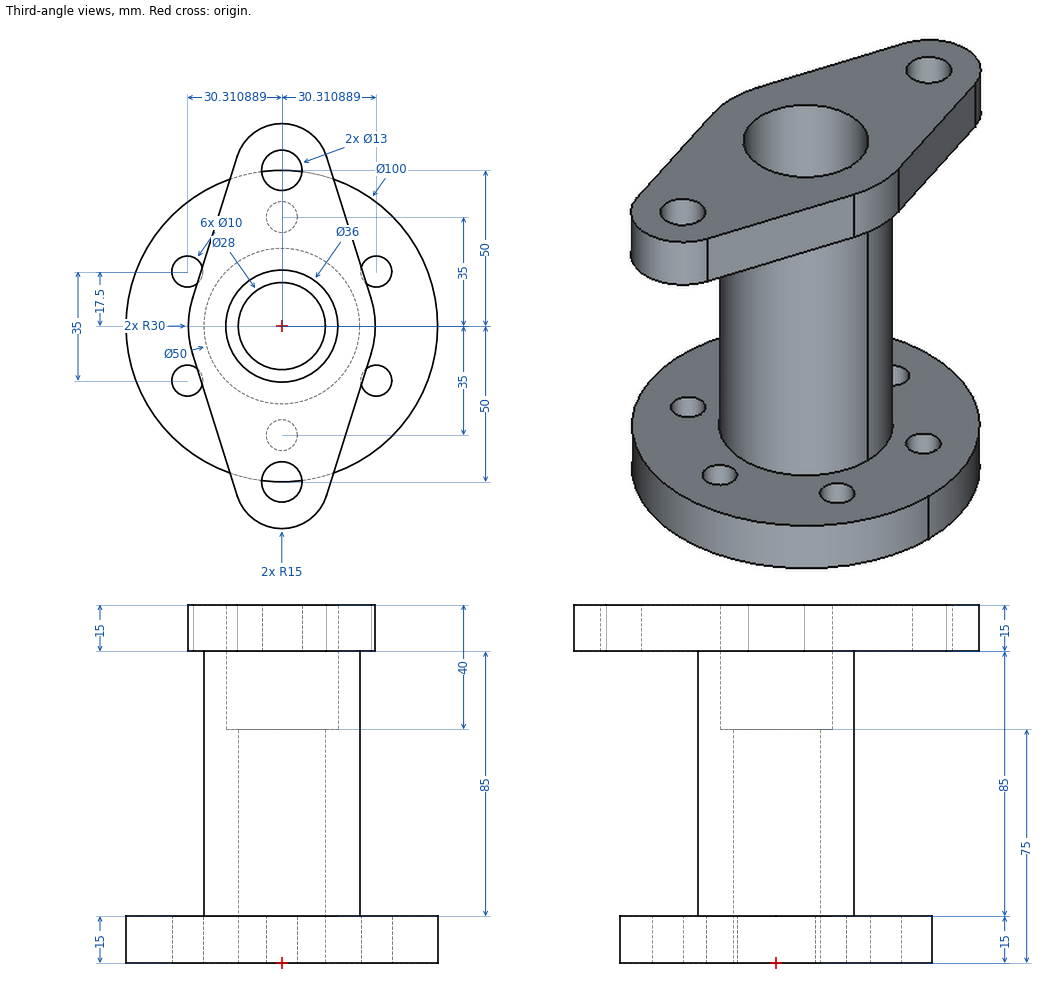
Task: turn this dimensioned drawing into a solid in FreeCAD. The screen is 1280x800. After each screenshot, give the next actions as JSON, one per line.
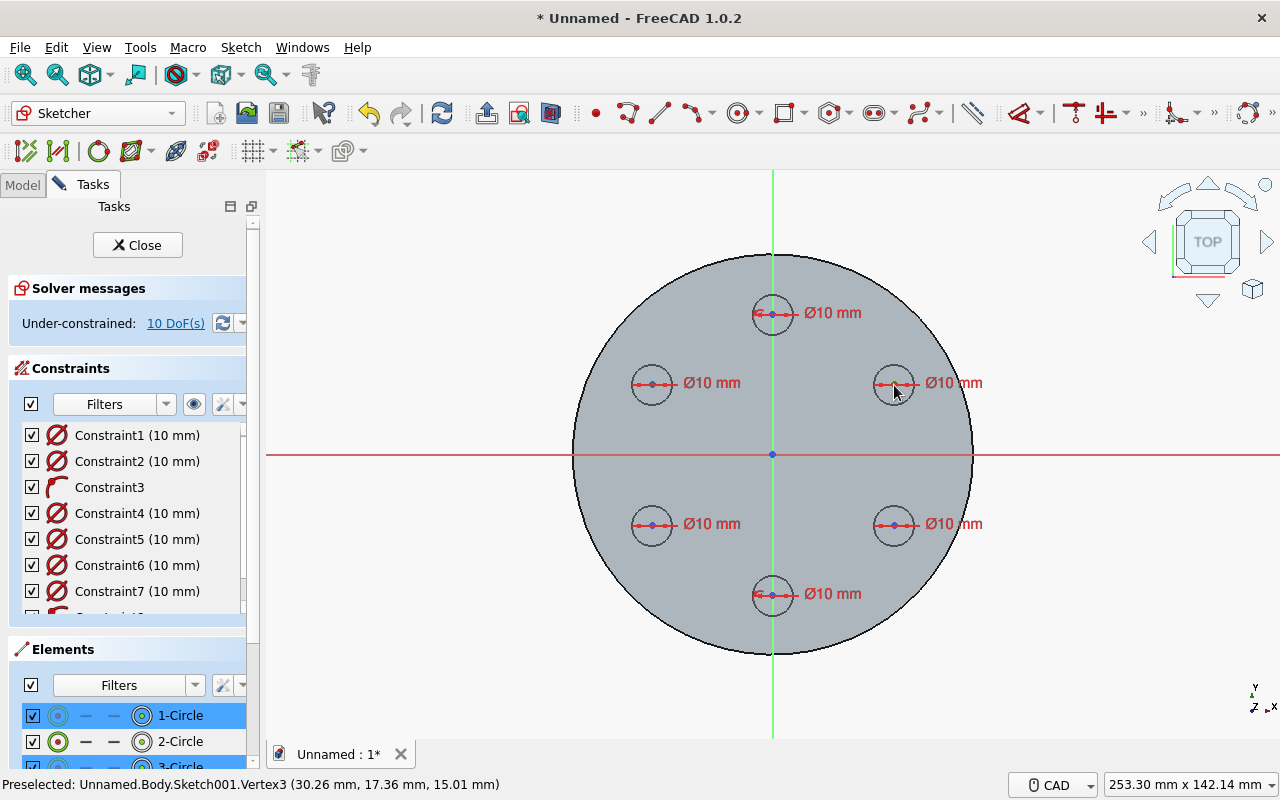
{"action": "key", "text": "h"}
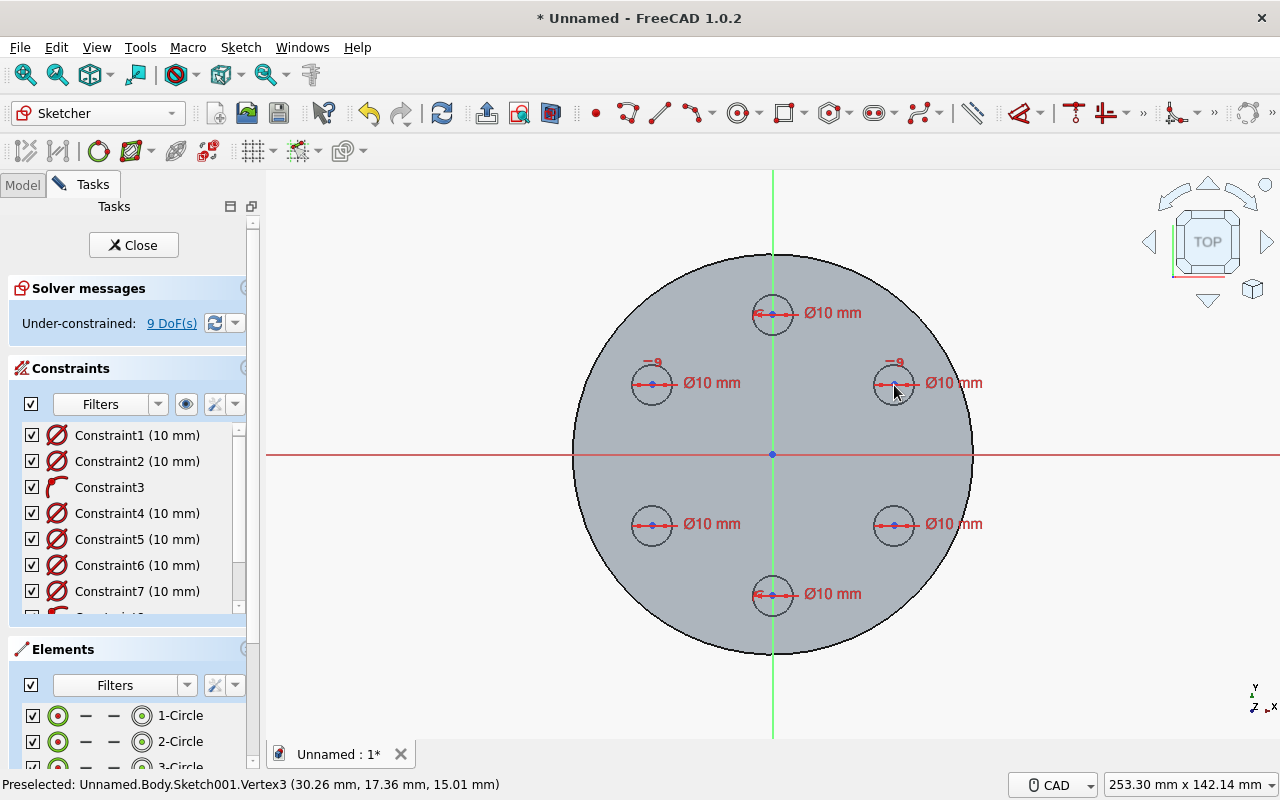
{"action": "left_click", "coordinate": [652, 385]}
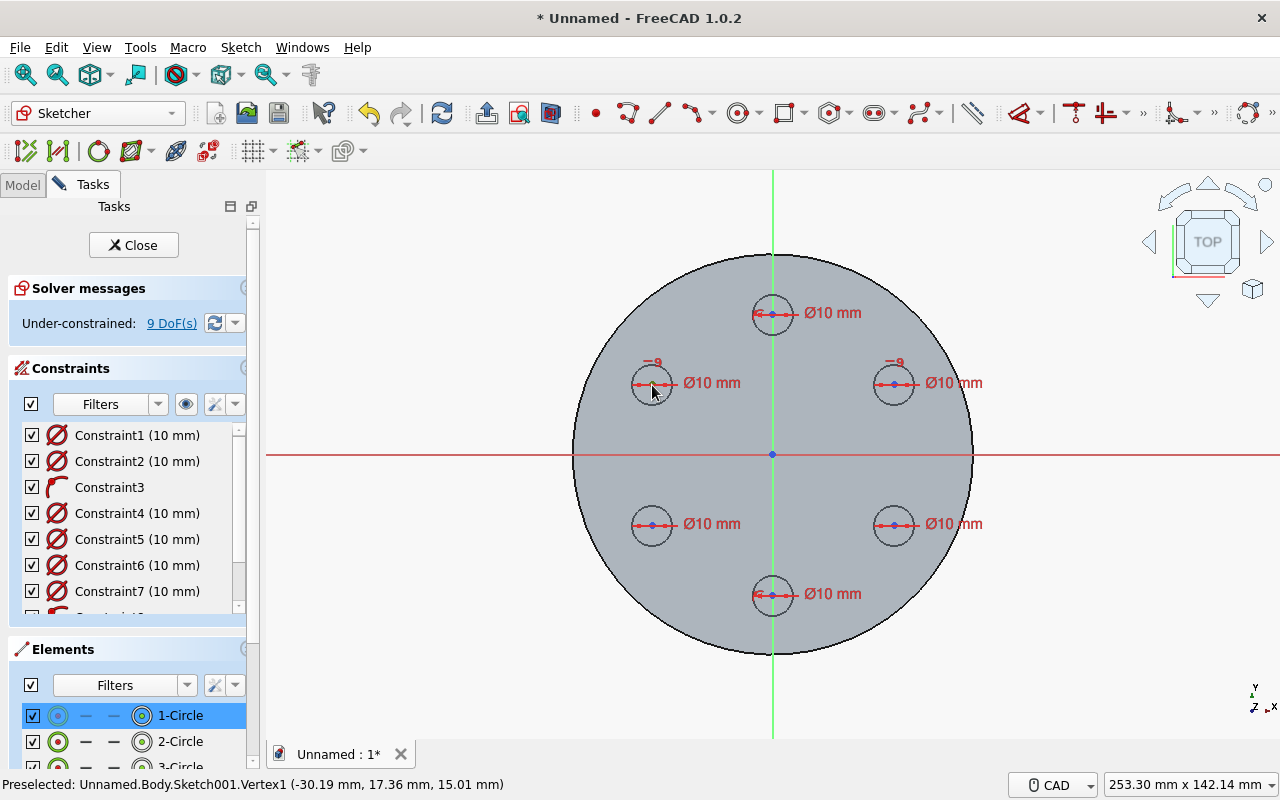
{"action": "left_click", "coordinate": [652, 526]}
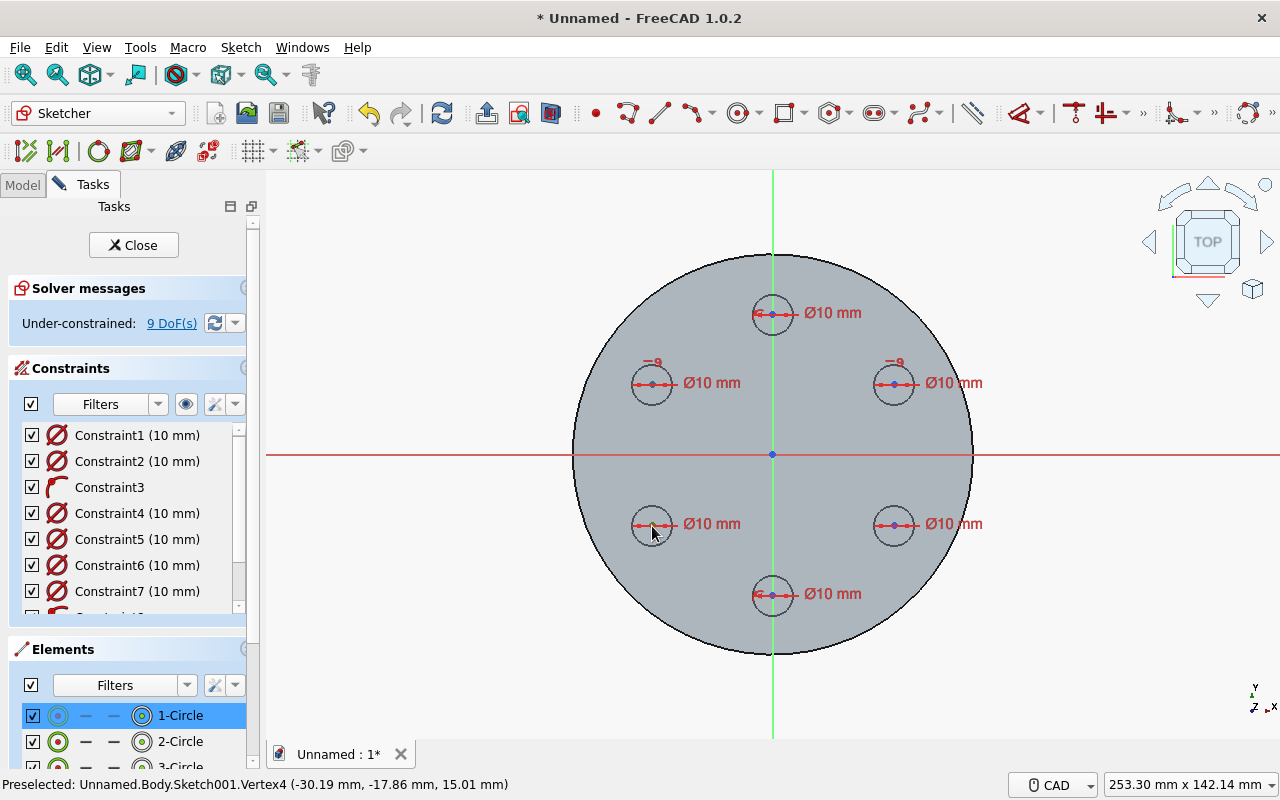
{"action": "key", "text": "v"}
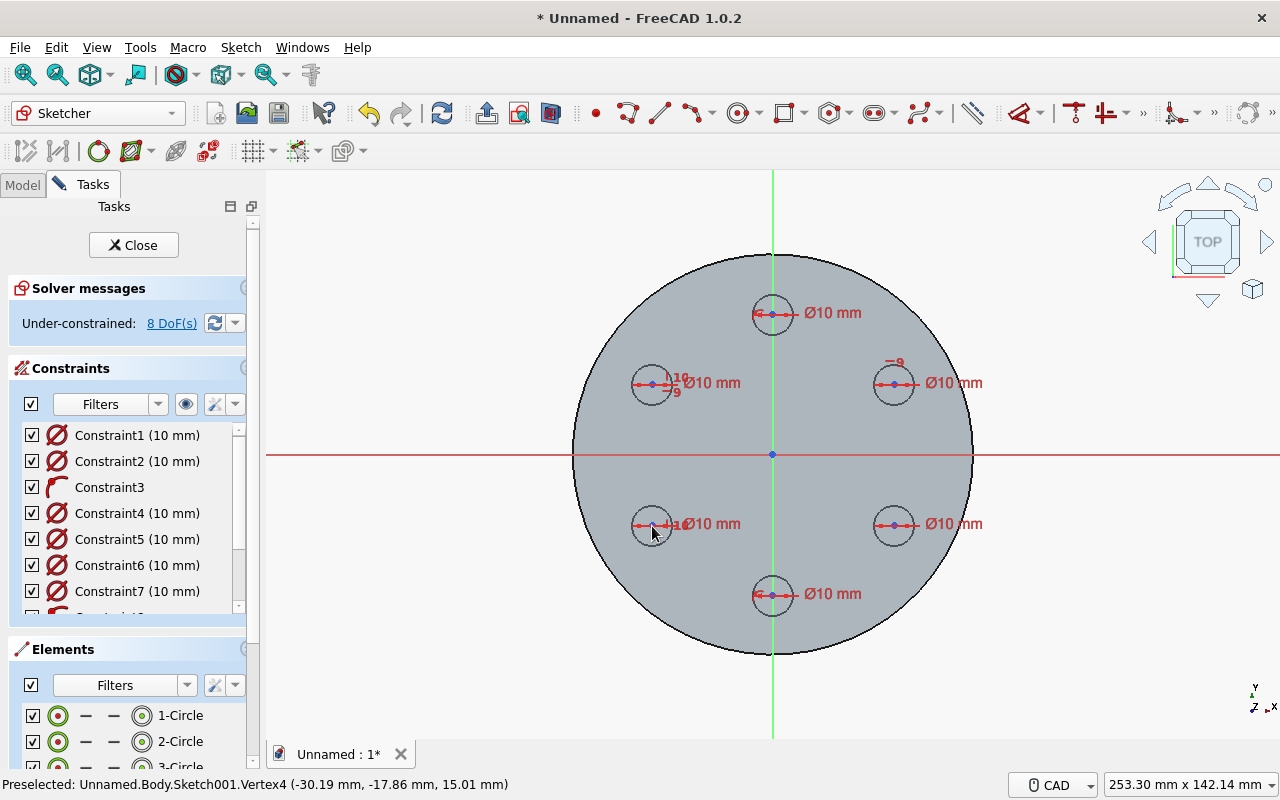
{"action": "left_click", "coordinate": [894, 385]}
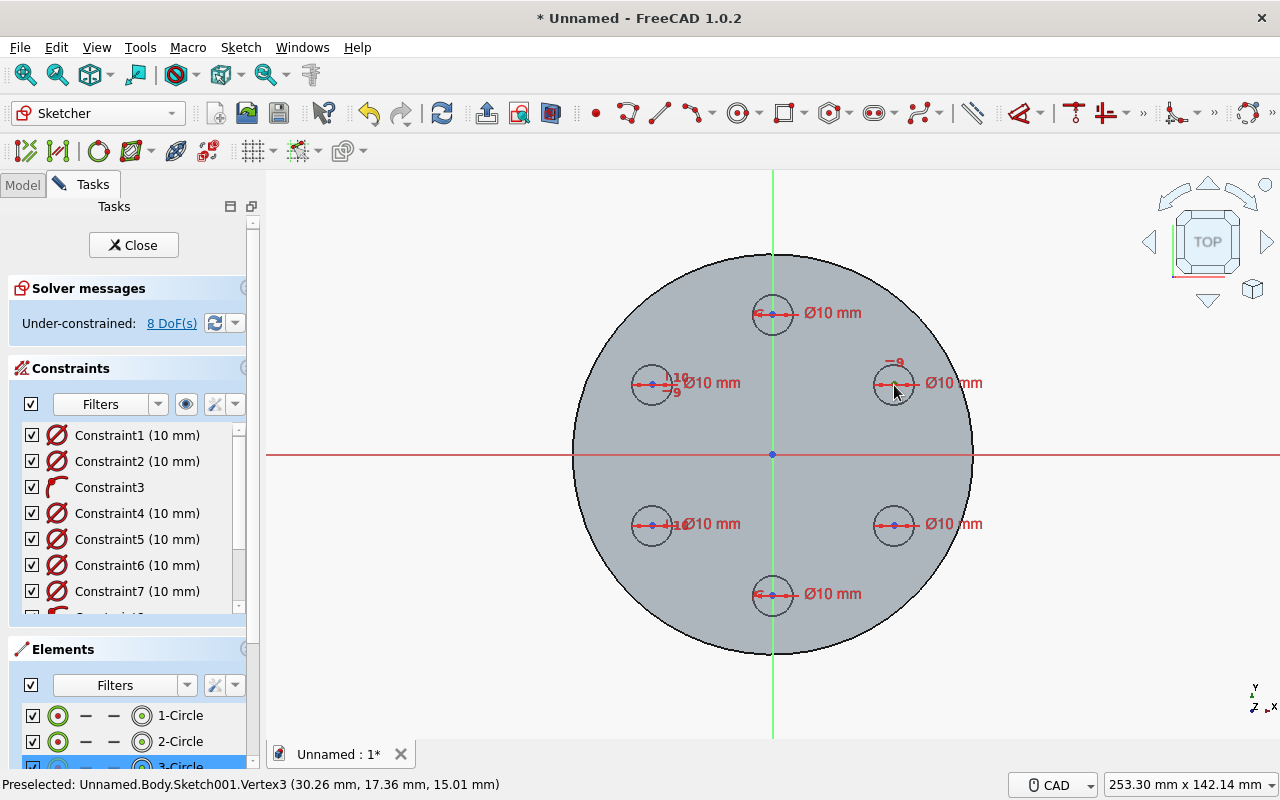
{"action": "left_click", "coordinate": [894, 526]}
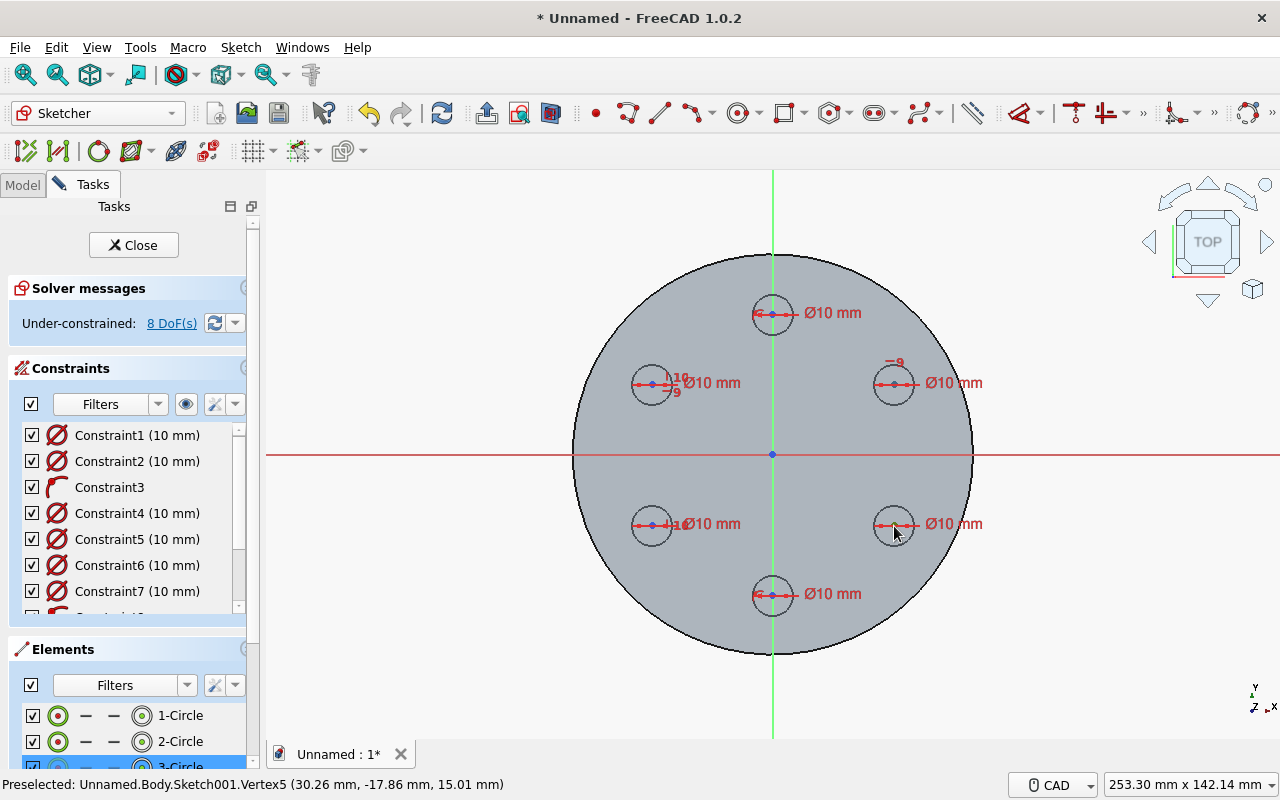
{"action": "key", "text": "v"}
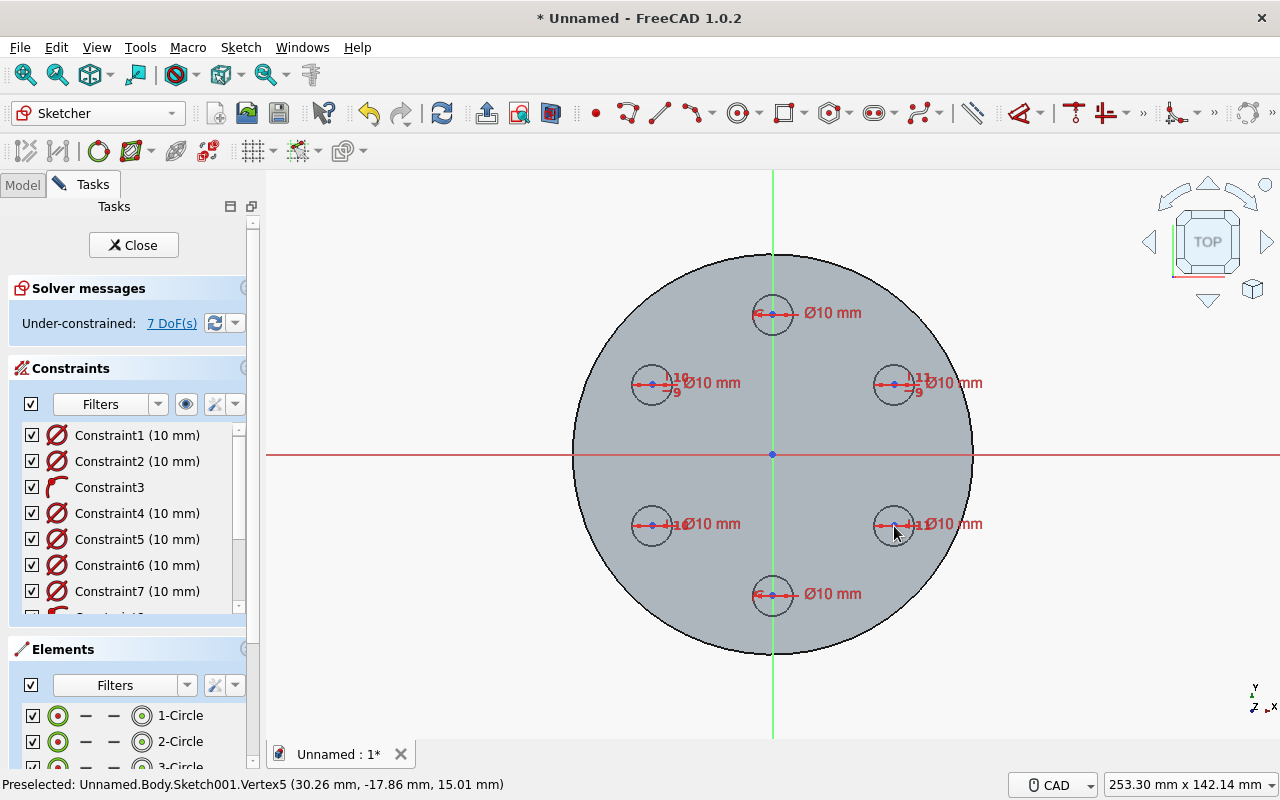
{"action": "left_click", "coordinate": [652, 526]}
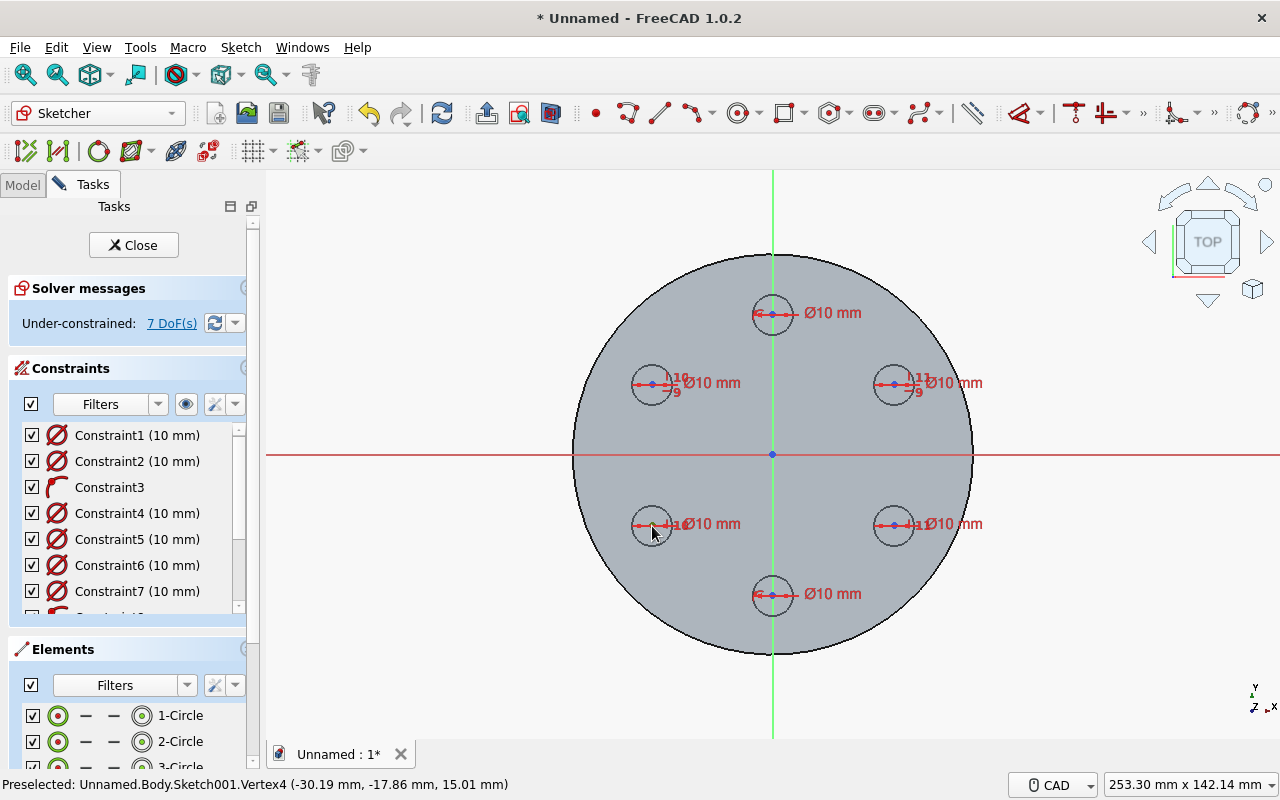
{"action": "left_click", "coordinate": [894, 526]}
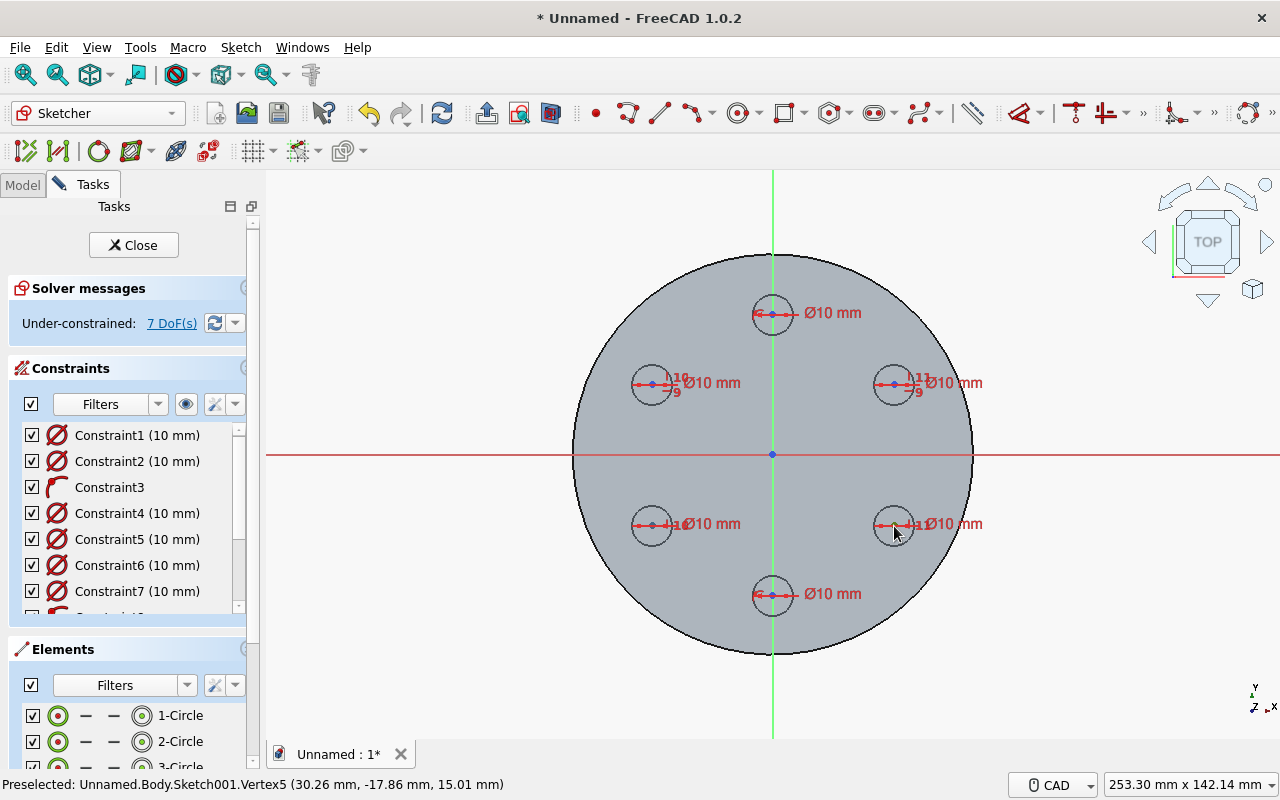
{"action": "key", "text": "h"}